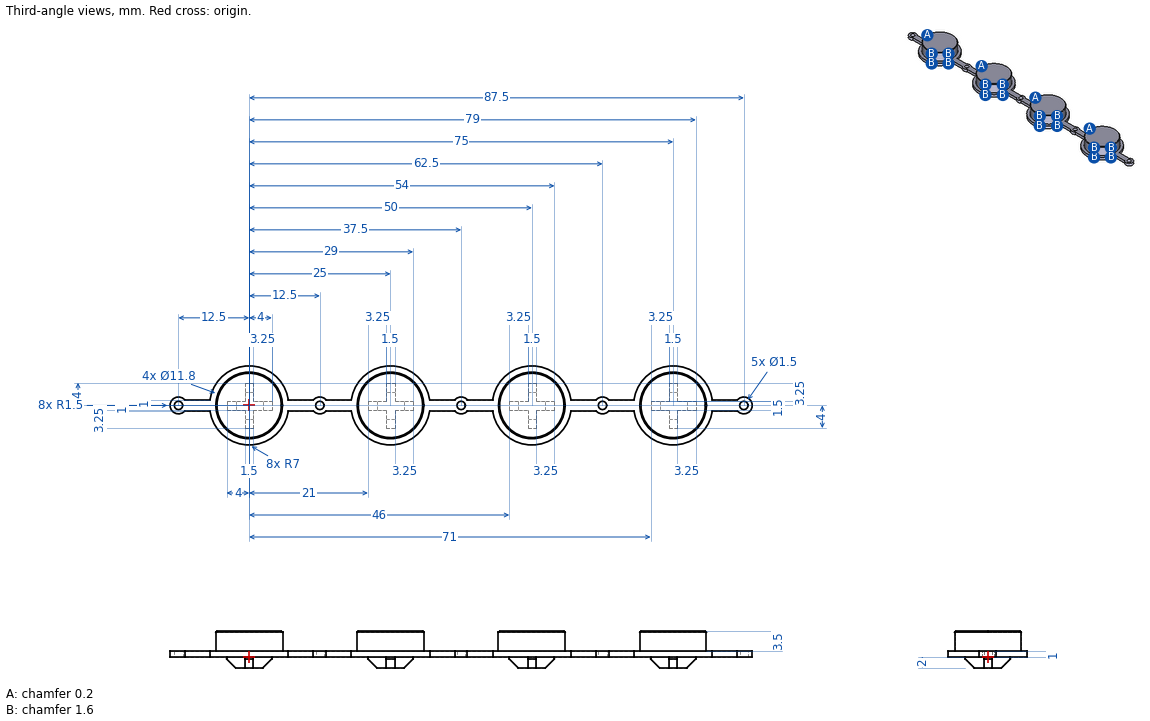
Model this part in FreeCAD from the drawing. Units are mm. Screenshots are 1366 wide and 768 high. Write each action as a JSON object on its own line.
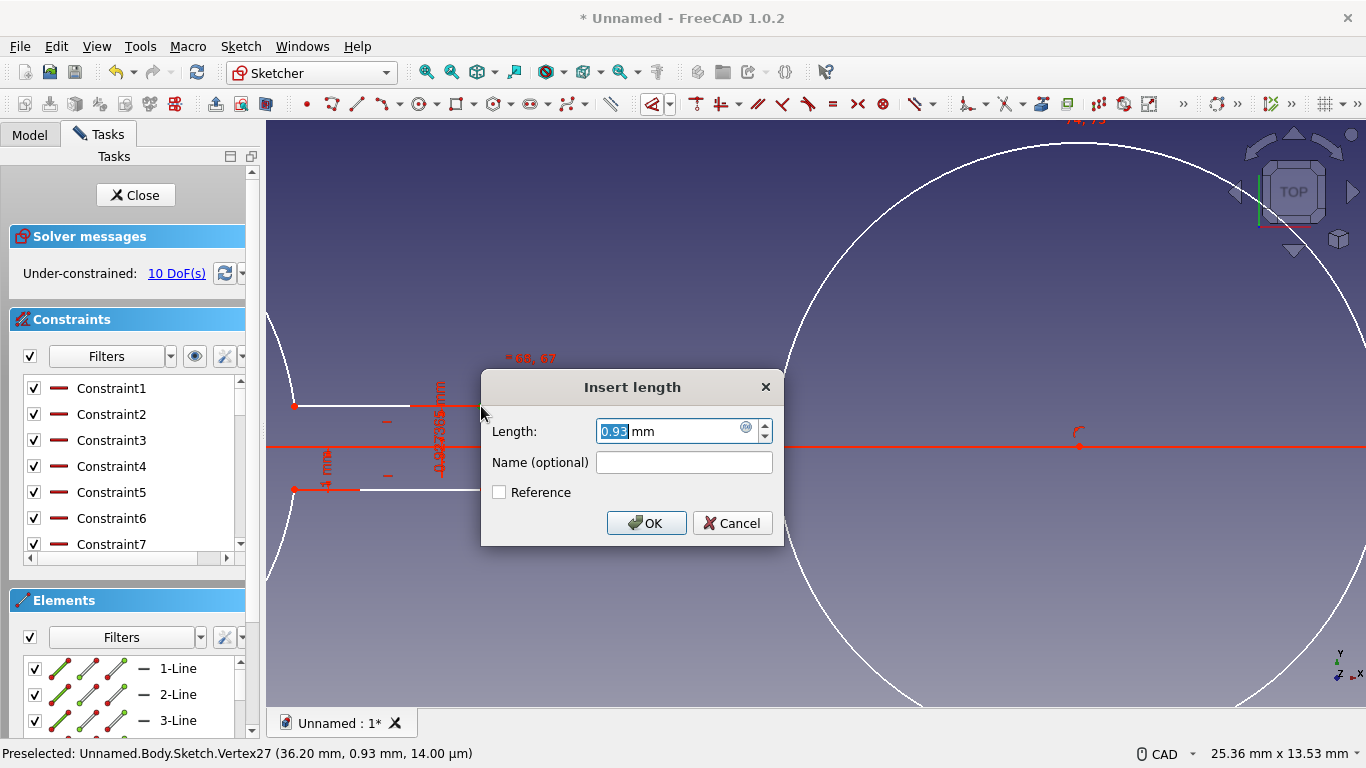
{"action": "type", "text": "1"}
{"action": "key", "text": "Return"}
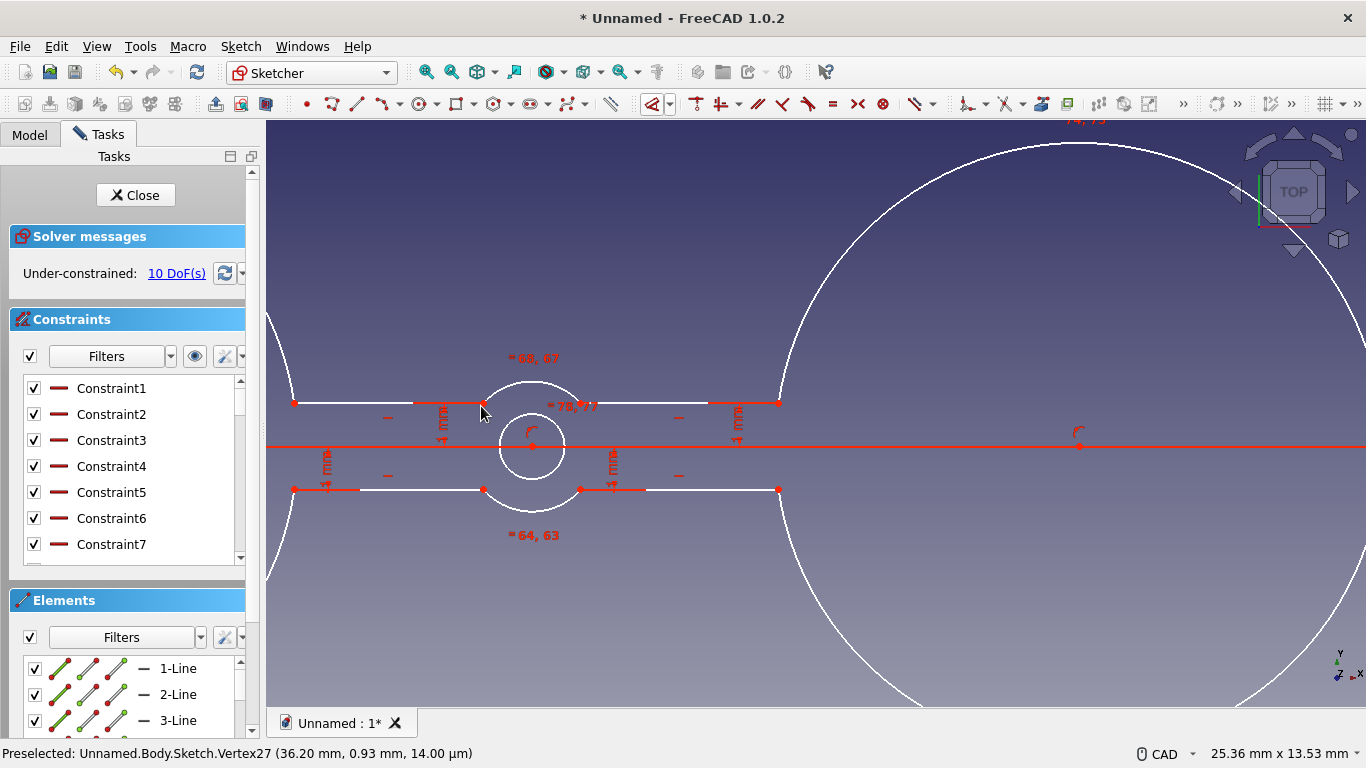
{"action": "scroll", "coordinate": [780, 408], "scroll_direction": "down", "scroll_amount": 10}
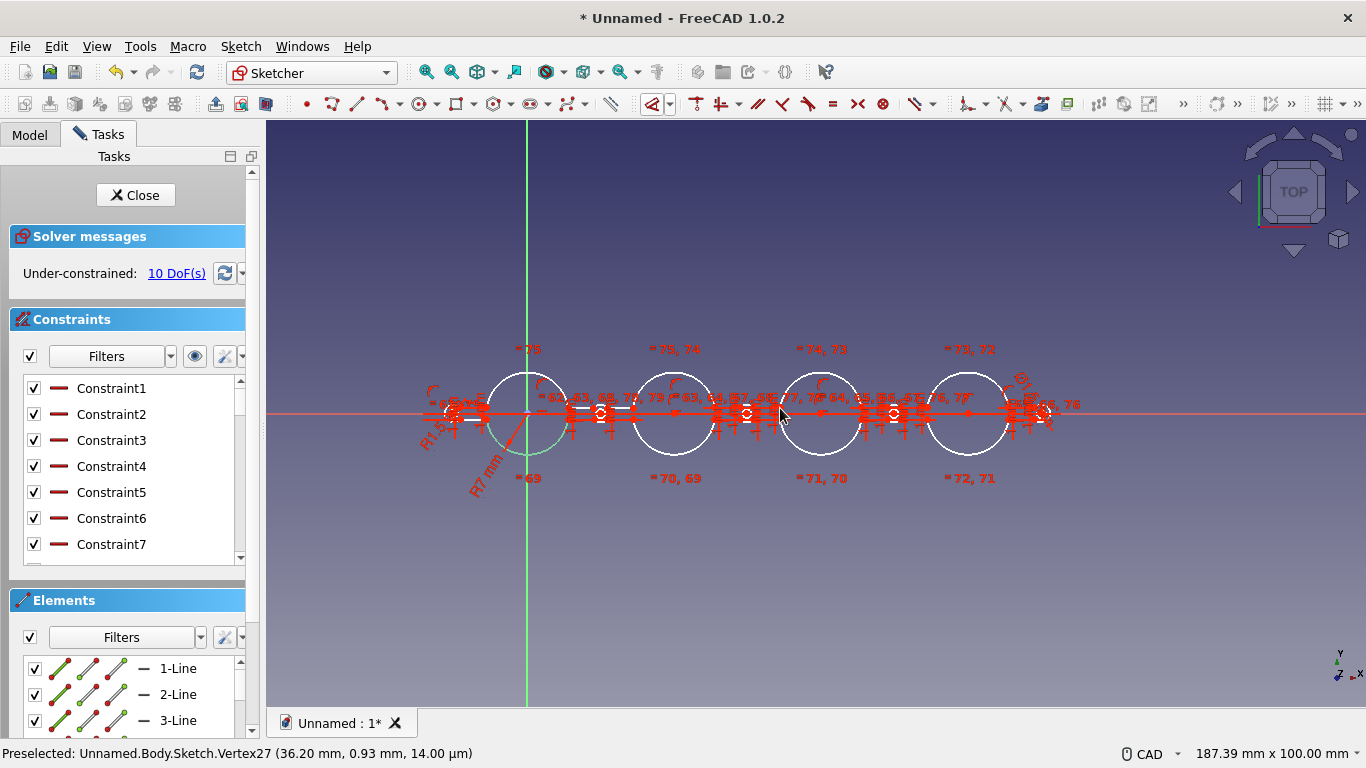
{"action": "scroll", "coordinate": [633, 408], "scroll_direction": "up", "scroll_amount": 10}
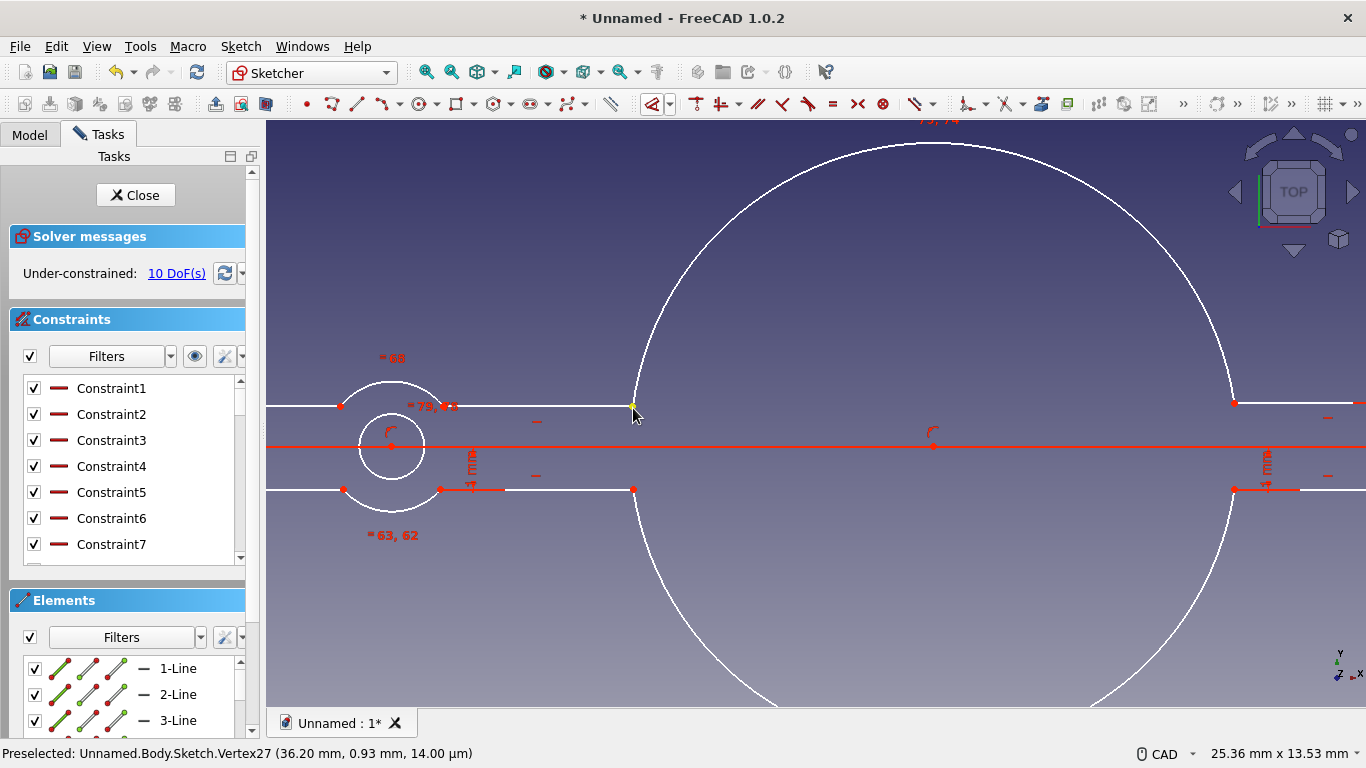
{"action": "left_click", "coordinate": [633, 406]}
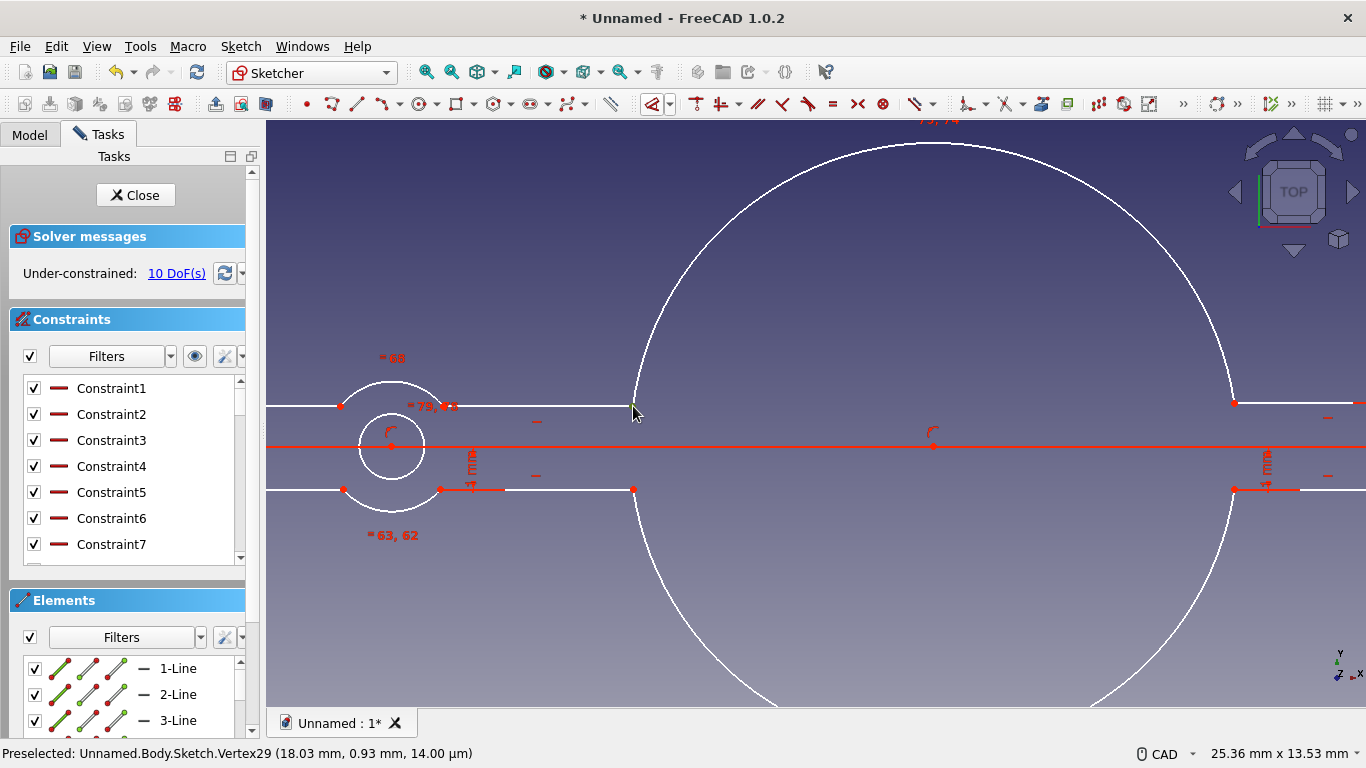
{"action": "key", "text": "i"}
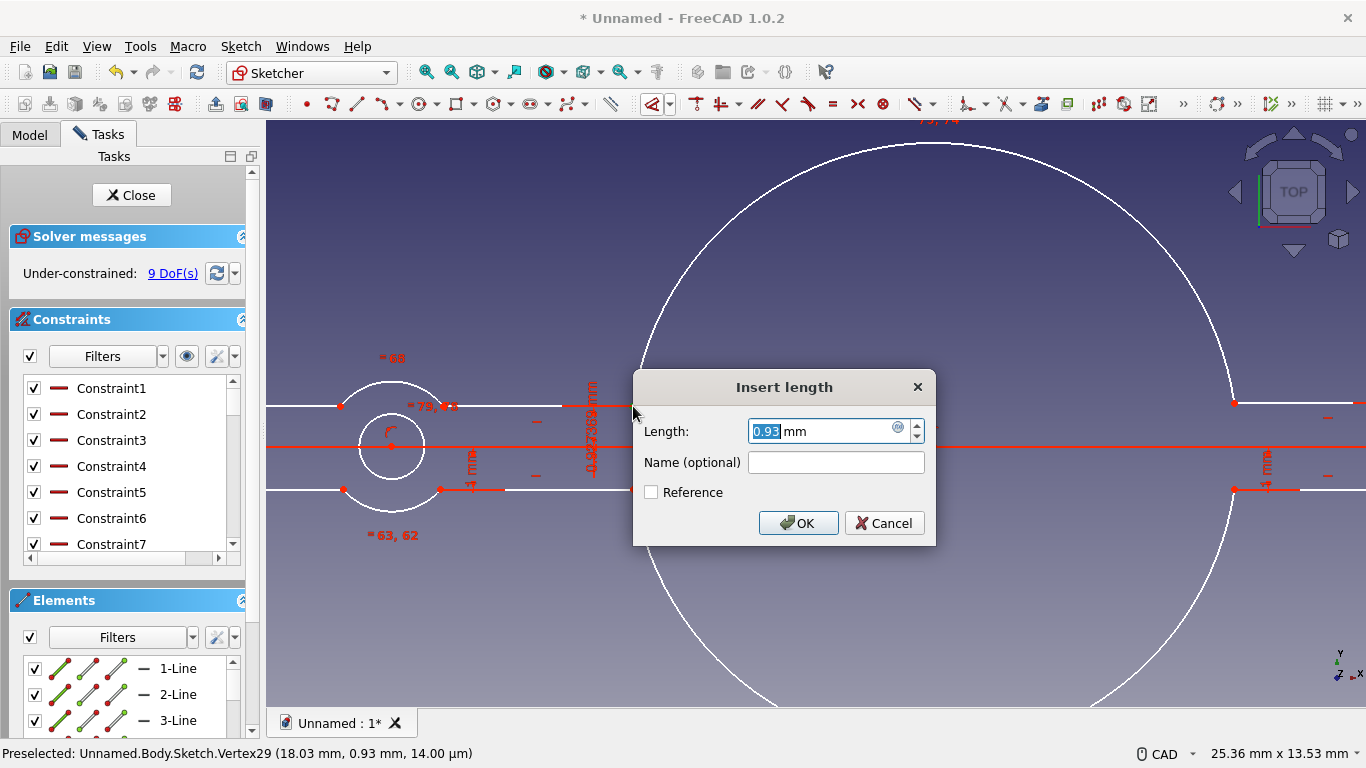
{"action": "type", "text": "1"}
{"action": "key", "text": "Return"}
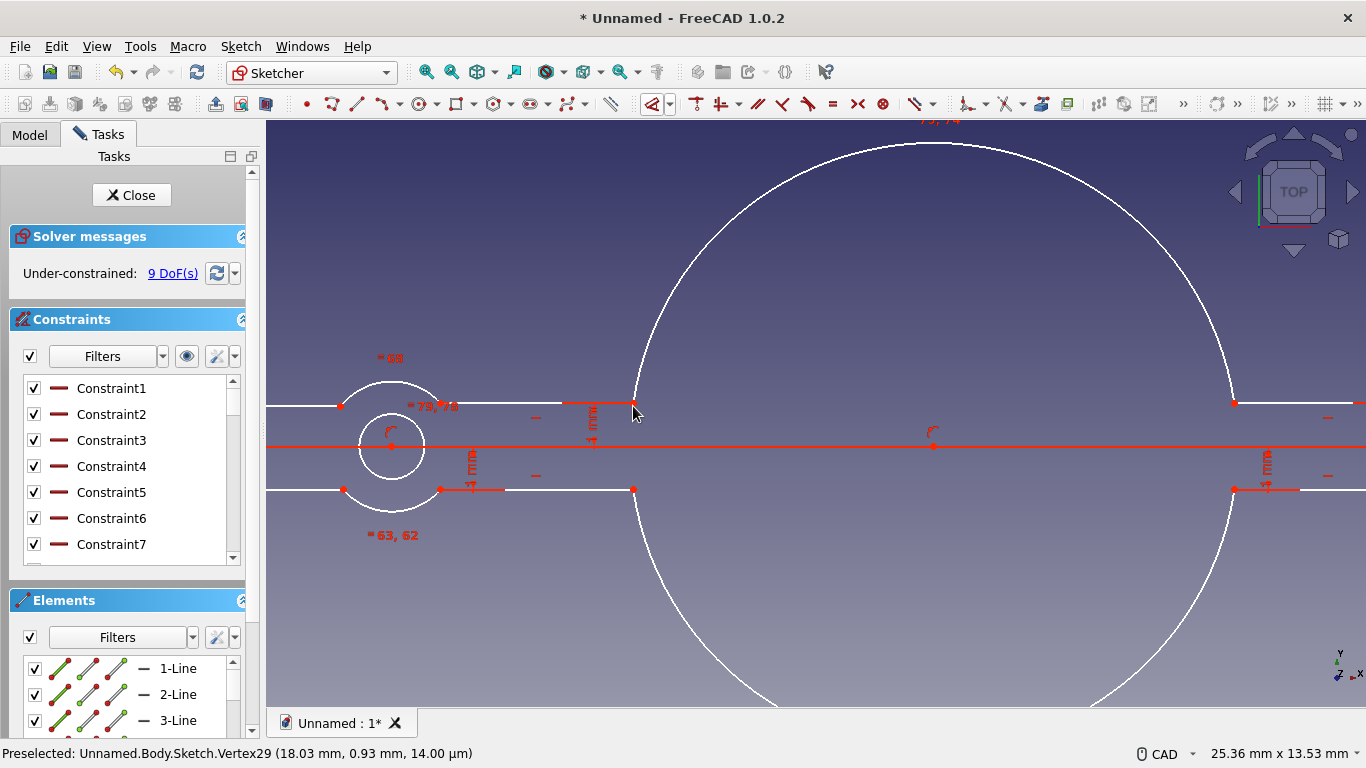
{"action": "left_click", "coordinate": [341, 406]}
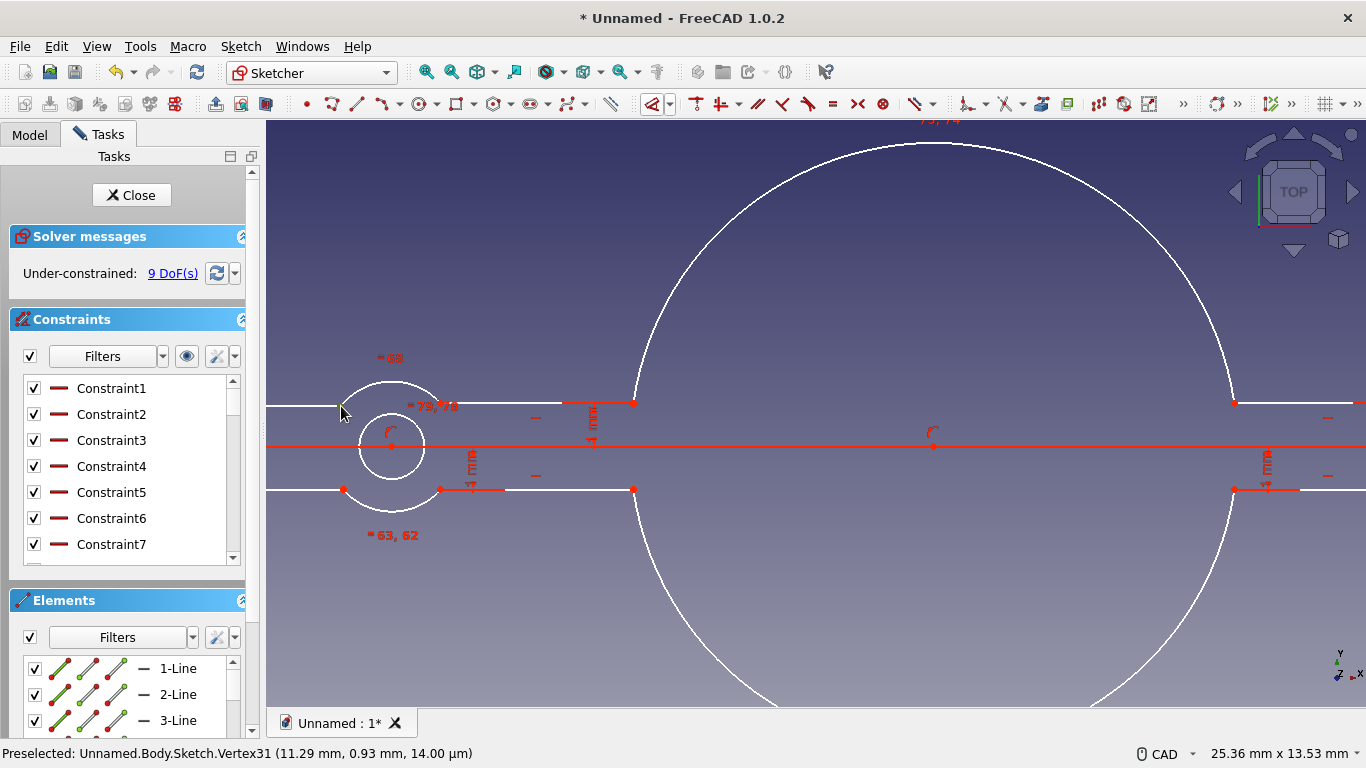
{"action": "left_click", "coordinate": [670, 104]}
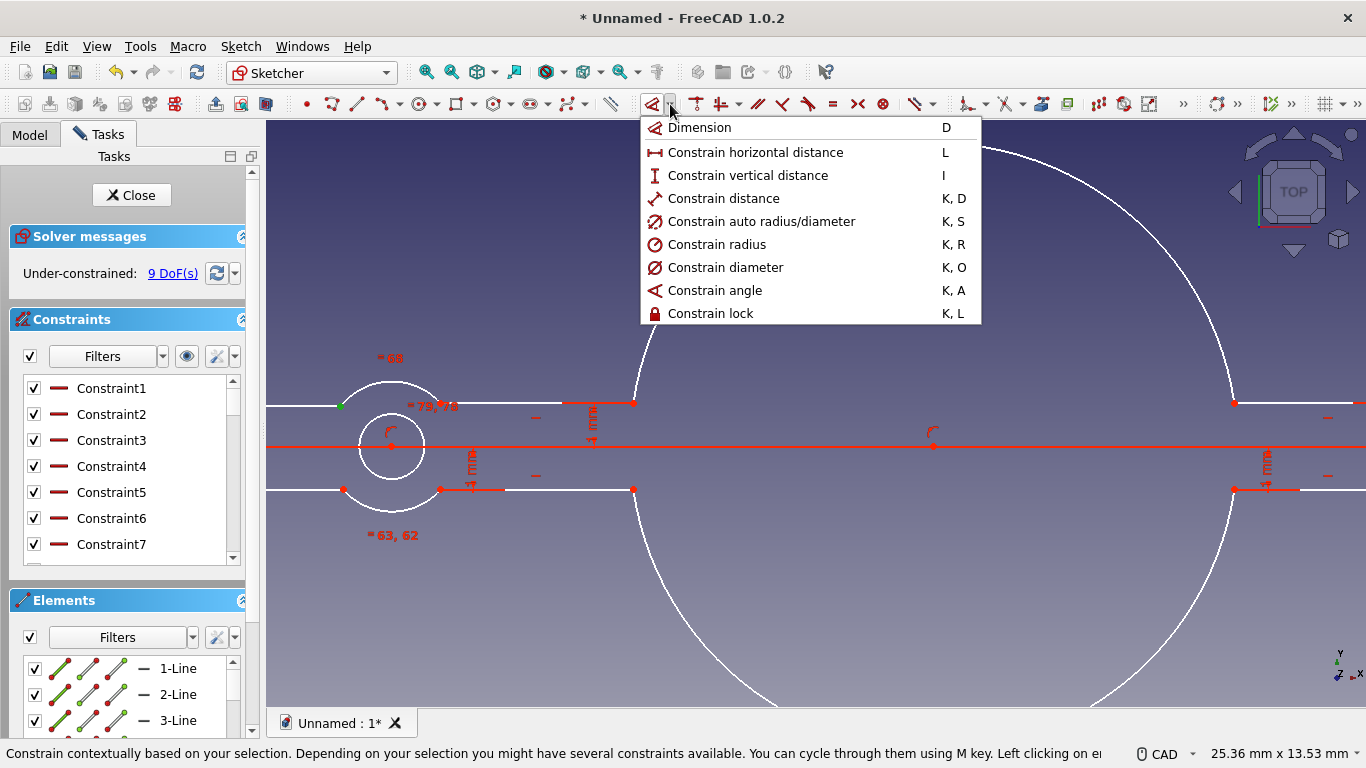
{"action": "left_click", "coordinate": [811, 176]}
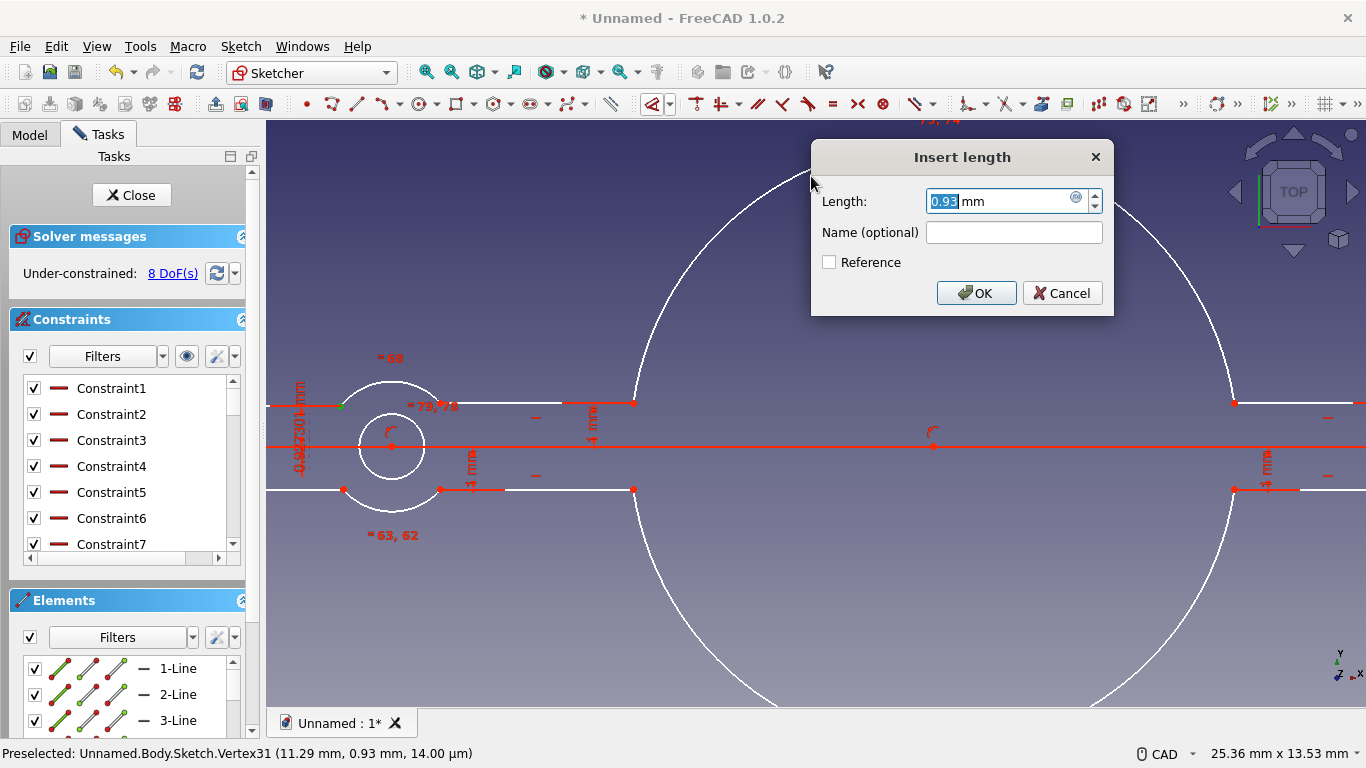
{"action": "type", "text": "1"}
{"action": "key", "text": "Return"}